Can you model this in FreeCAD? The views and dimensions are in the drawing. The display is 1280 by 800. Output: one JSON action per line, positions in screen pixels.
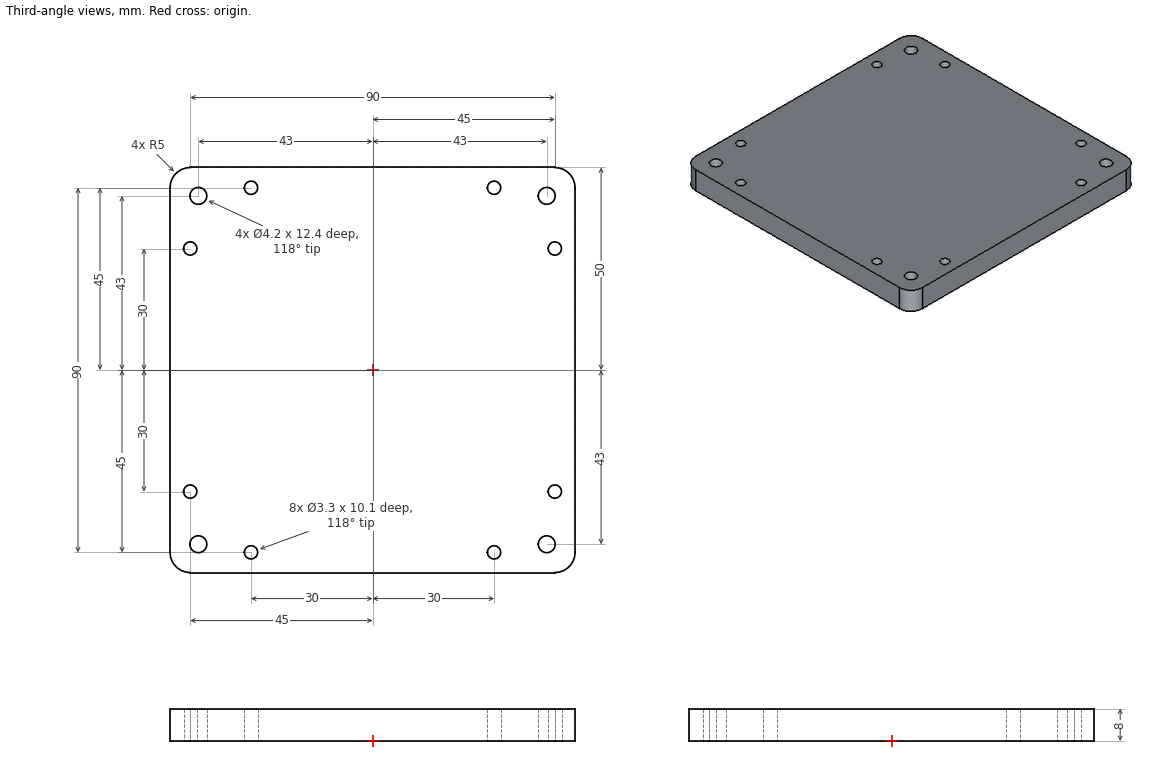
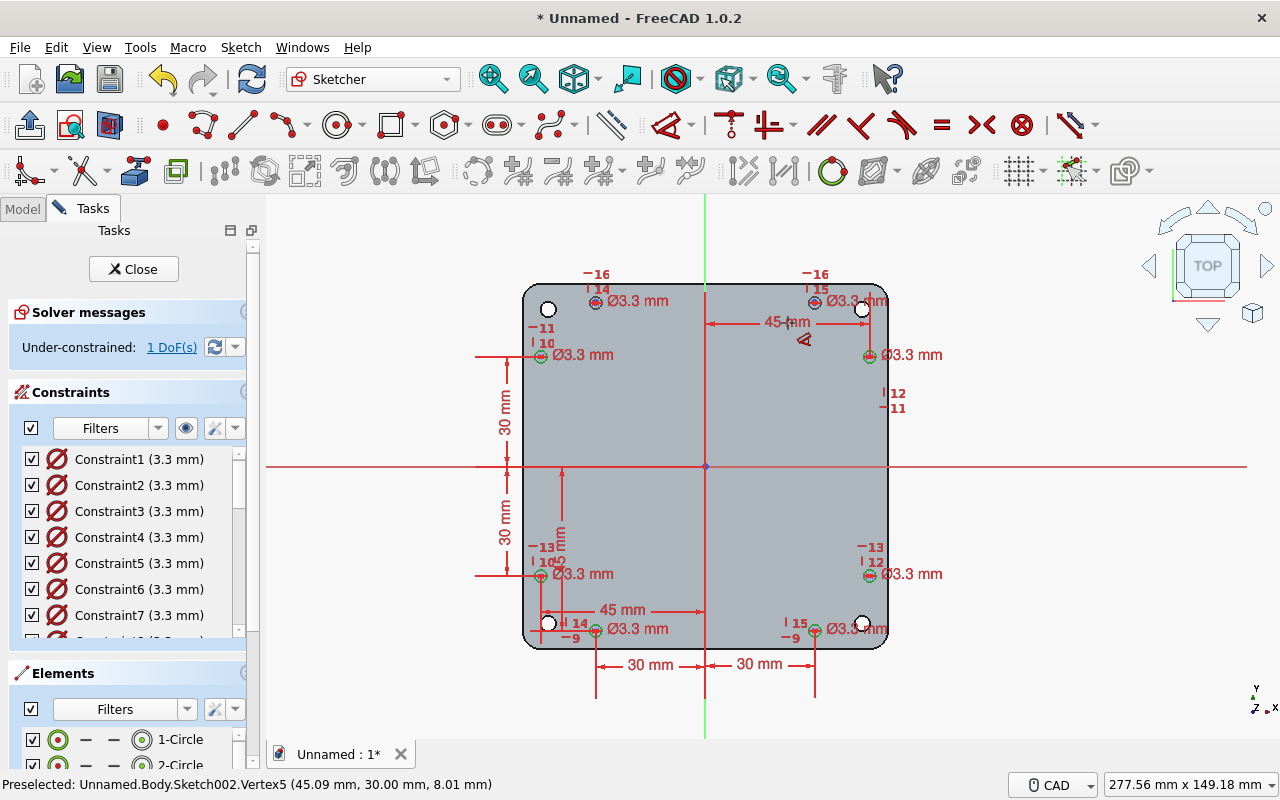
{"action": "left_click", "coordinate": [596, 303]}
{"action": "left_click", "coordinate": [562, 385]}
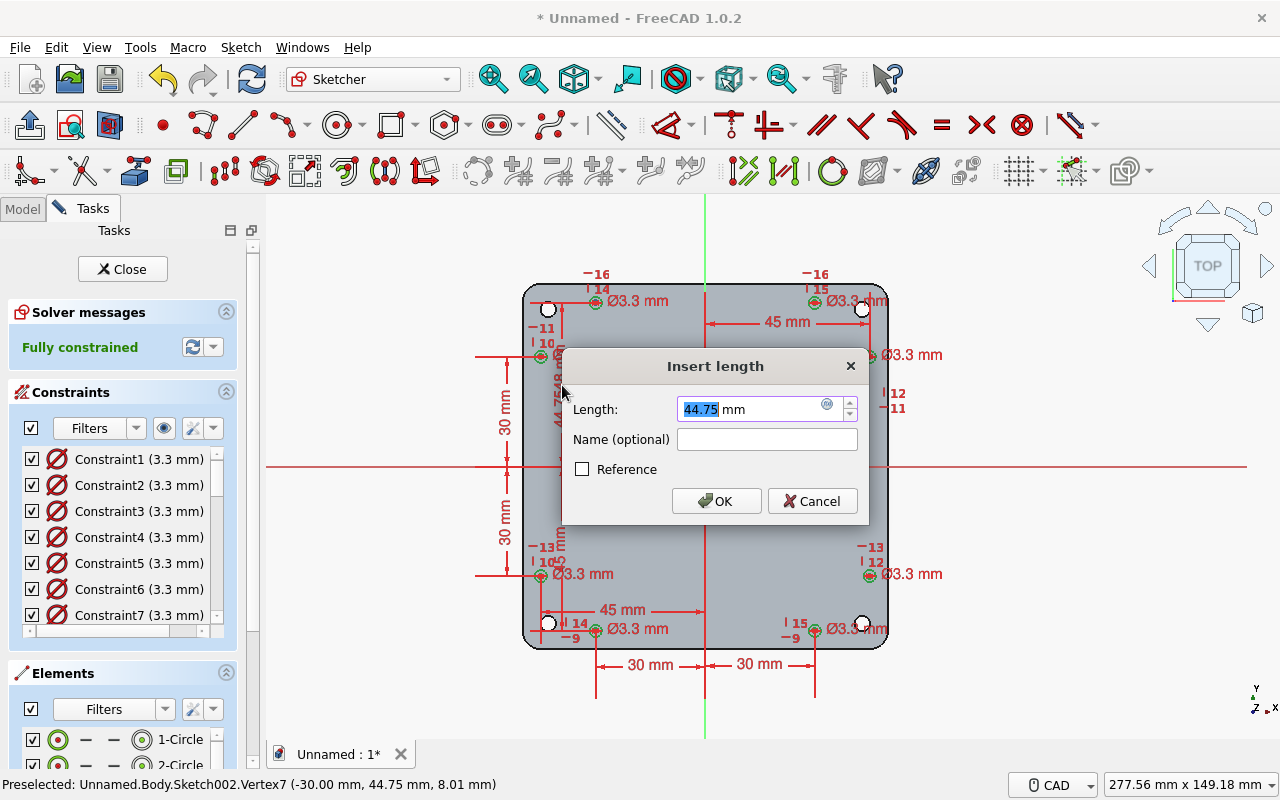
{"action": "type", "text": "45"}
{"action": "key", "text": "Return"}
{"action": "key", "text": "Escape"}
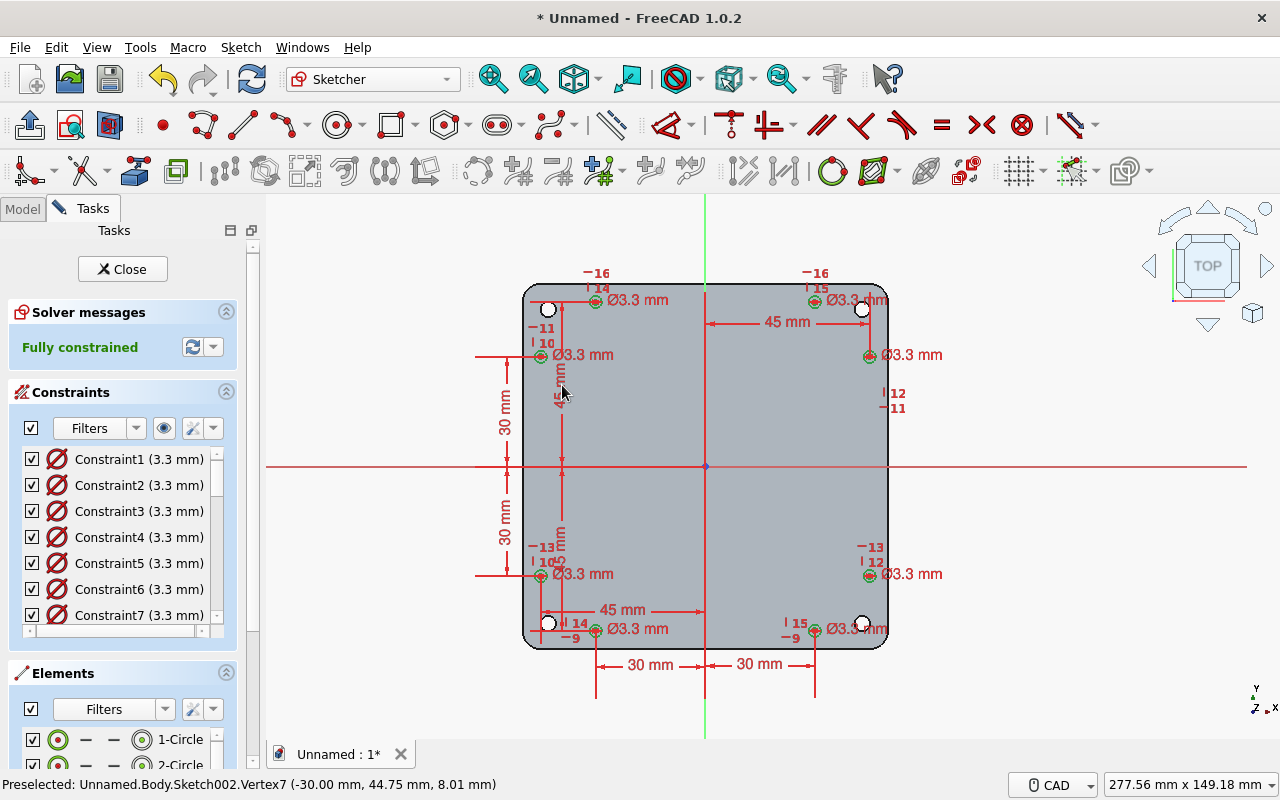
{"action": "left_click", "coordinate": [123, 269]}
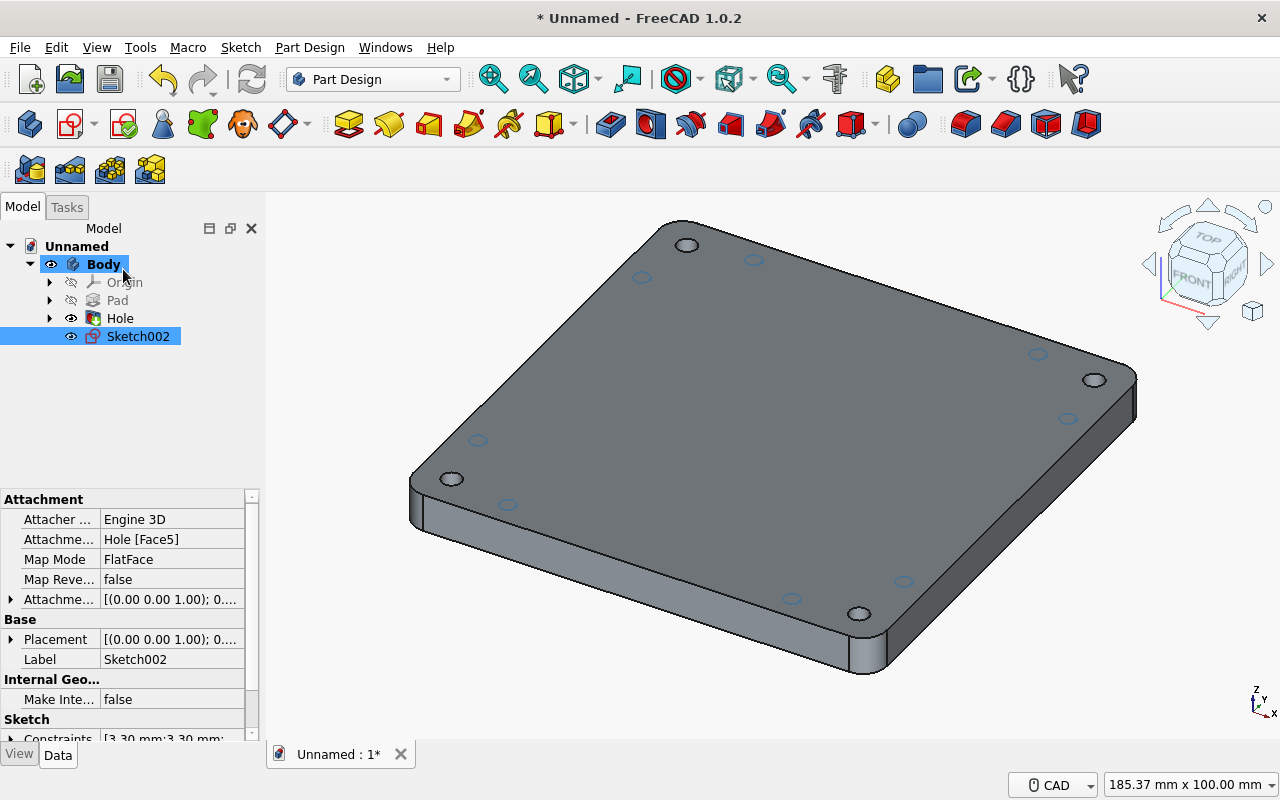
{"action": "left_click", "coordinate": [652, 124]}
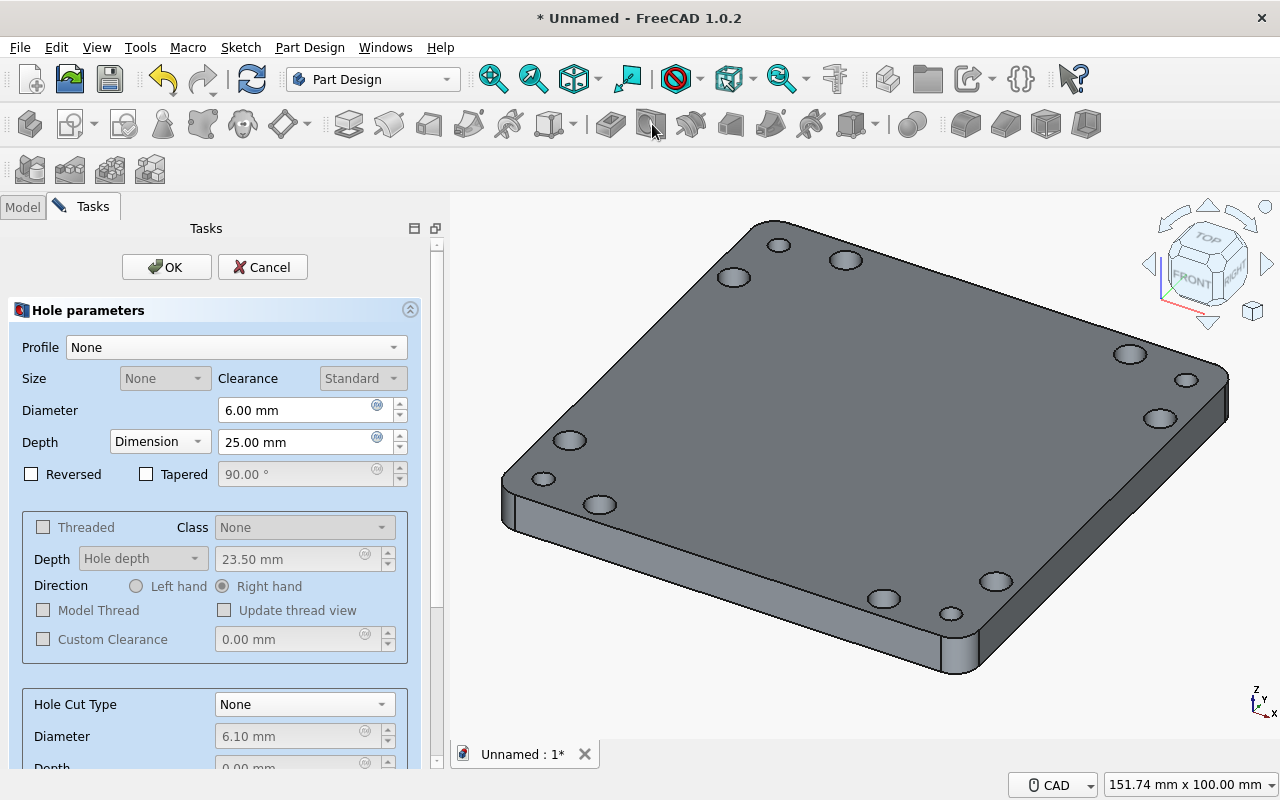
{"action": "triple_click", "coordinate": [305, 410]}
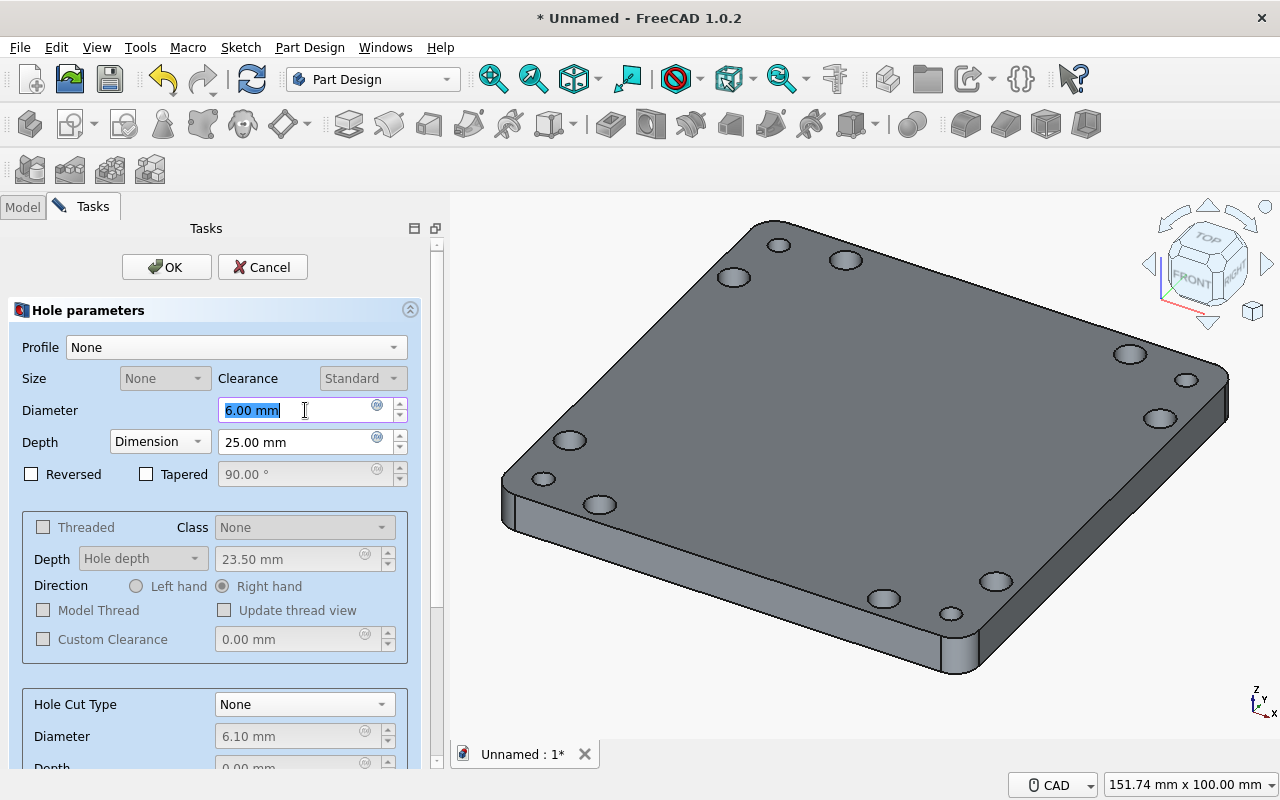
{"action": "type", "text": "3.3"}
{"action": "key", "text": "Tab"}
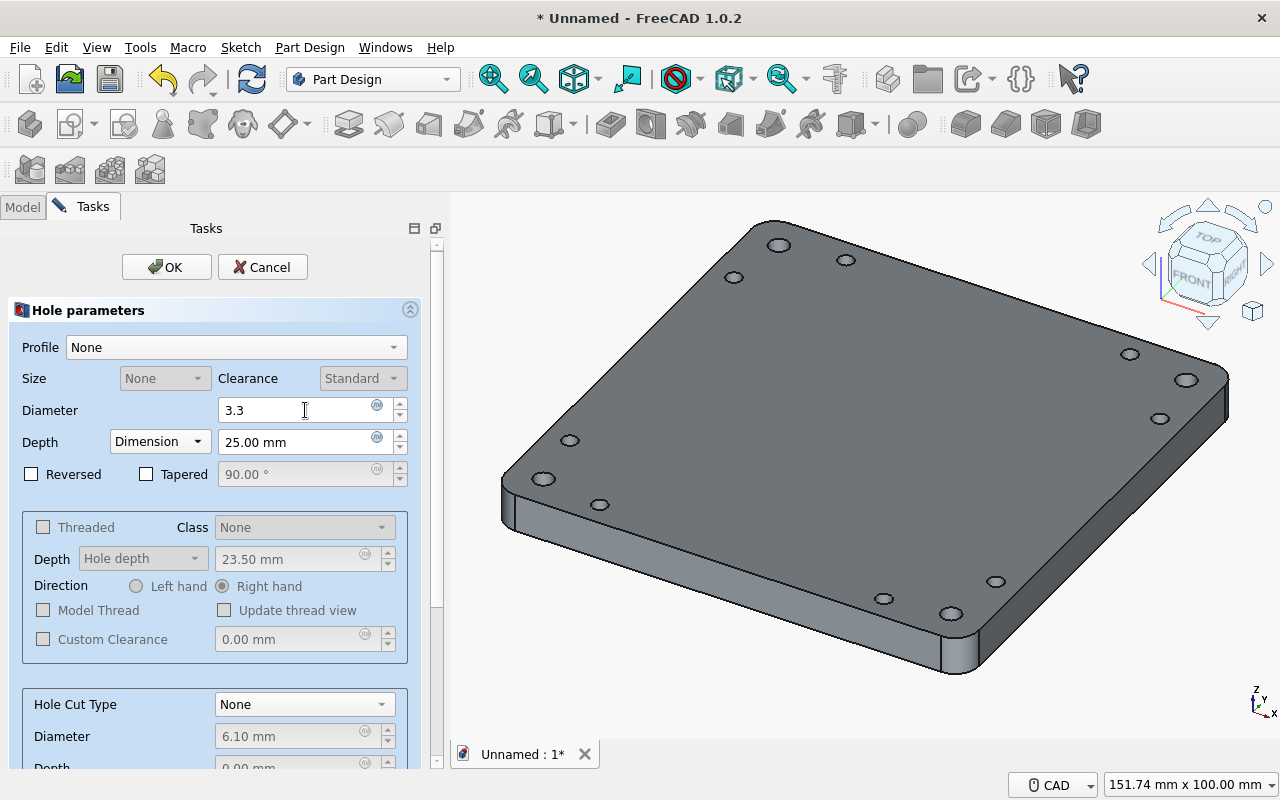
{"action": "triple_click", "coordinate": [305, 442]}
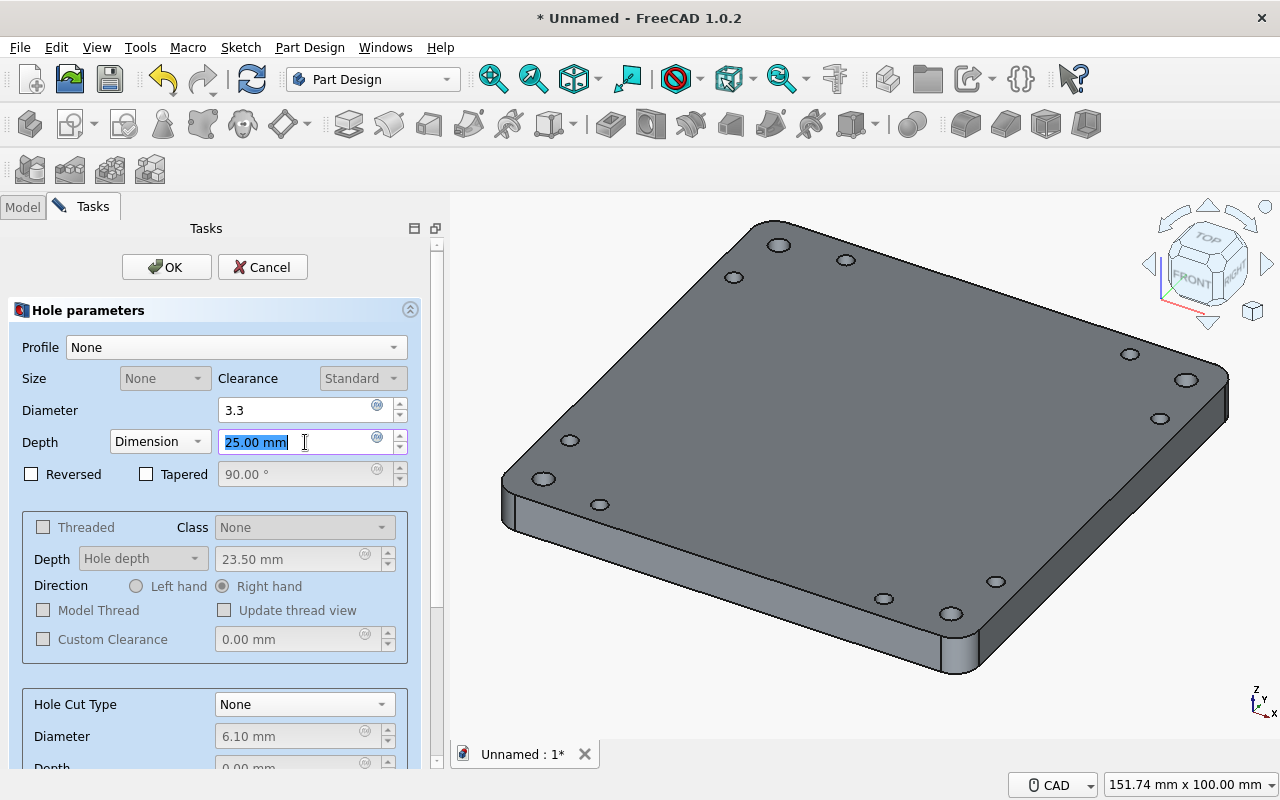
{"action": "type", "text": "10.1"}
{"action": "key", "text": "Tab"}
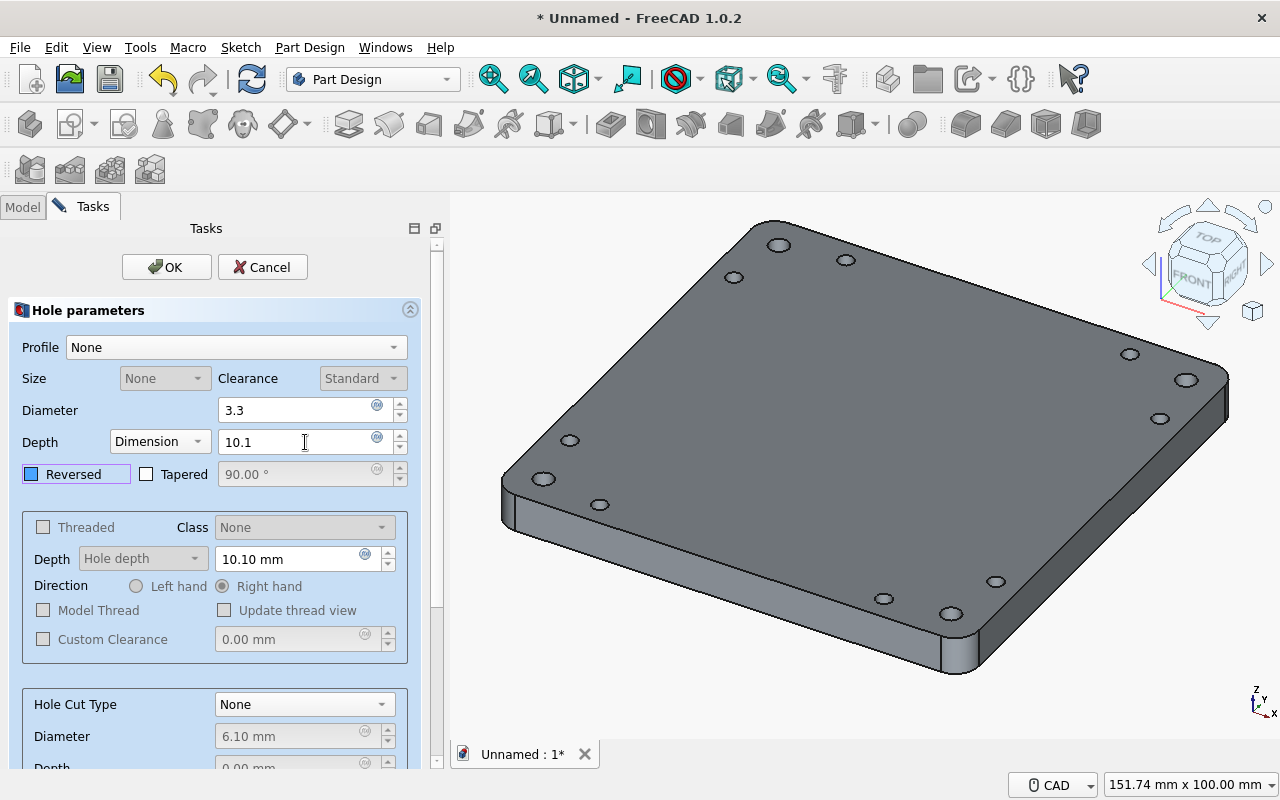
{"action": "left_click", "coordinate": [167, 267]}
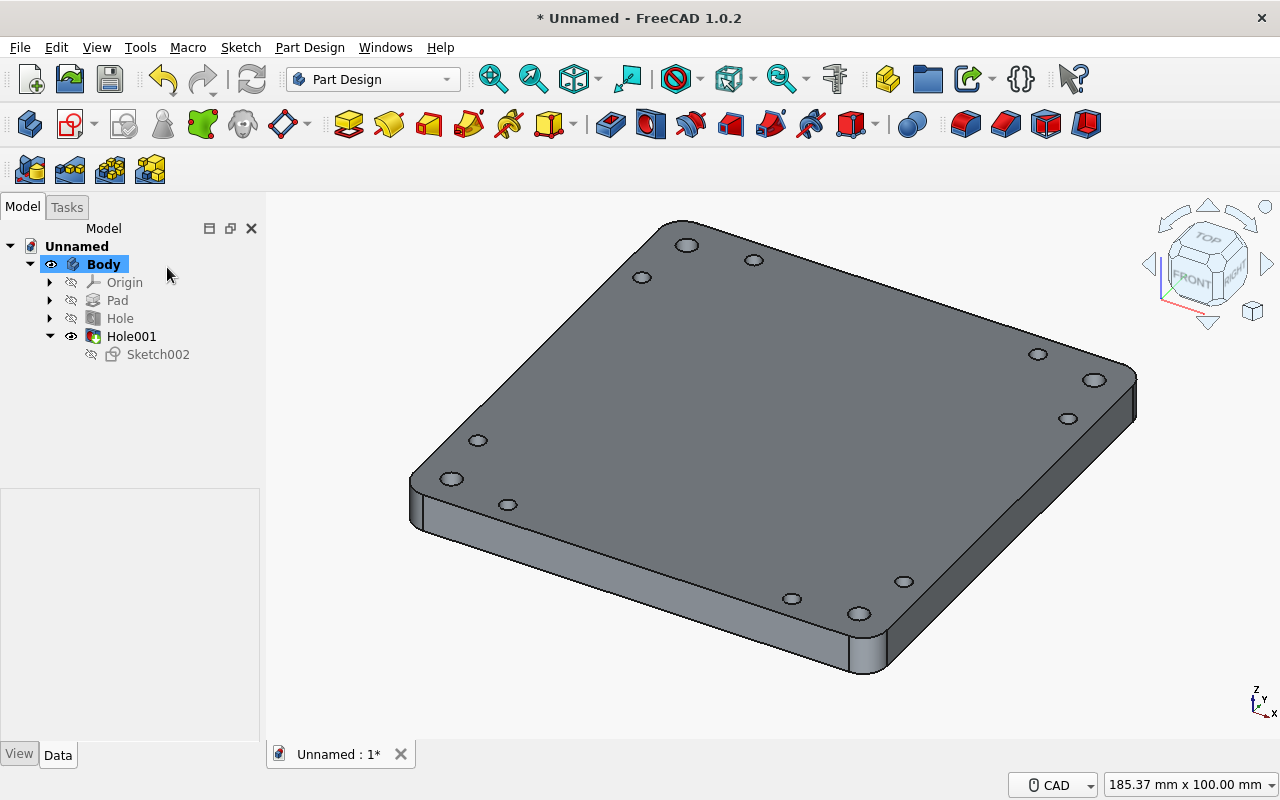
{"action": "key", "text": "0"}